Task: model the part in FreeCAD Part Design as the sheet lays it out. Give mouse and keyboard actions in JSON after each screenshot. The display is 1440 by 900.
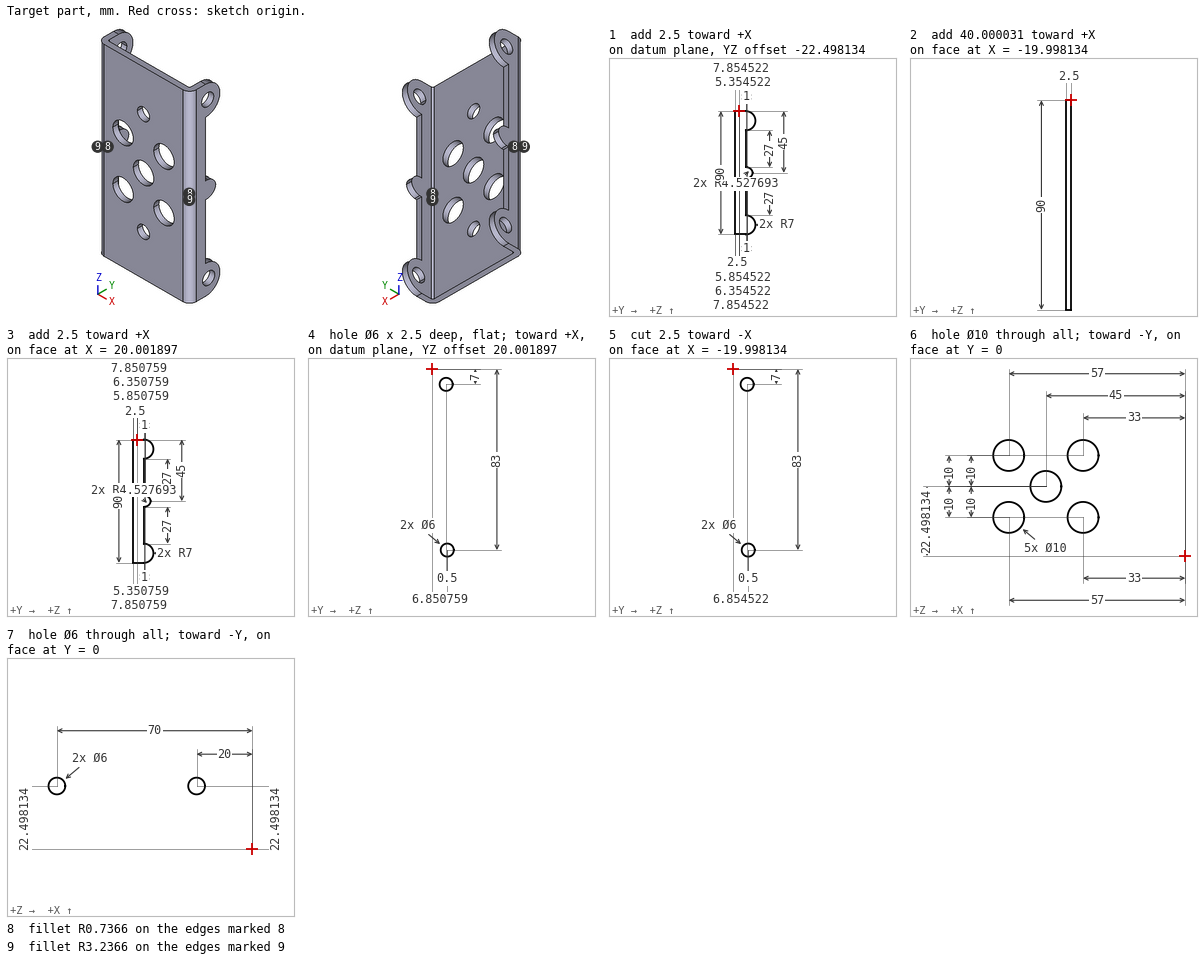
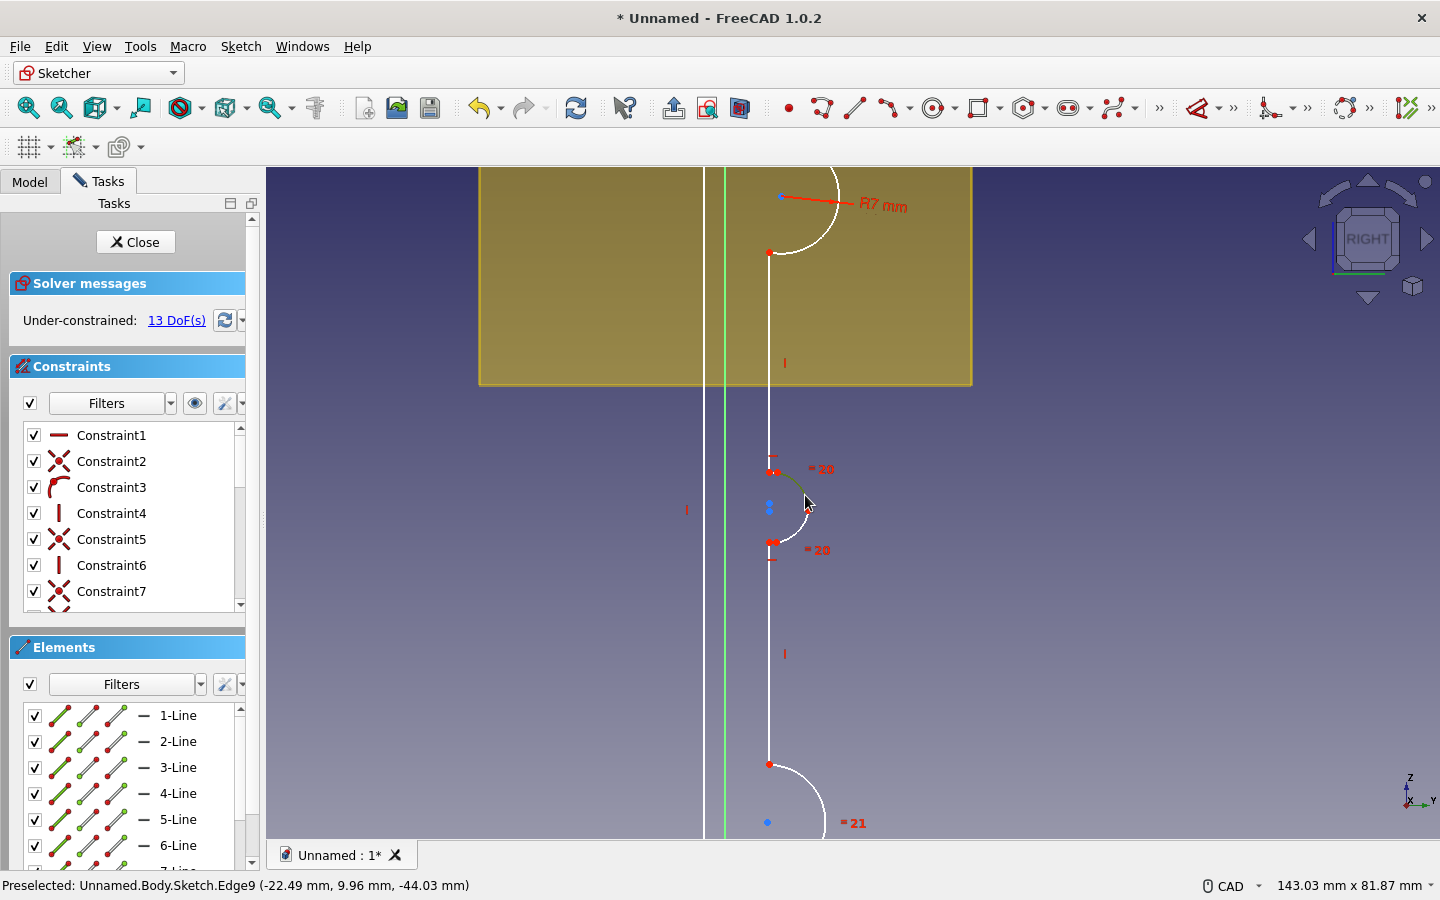
{"action": "left_click", "coordinate": [1218, 108]}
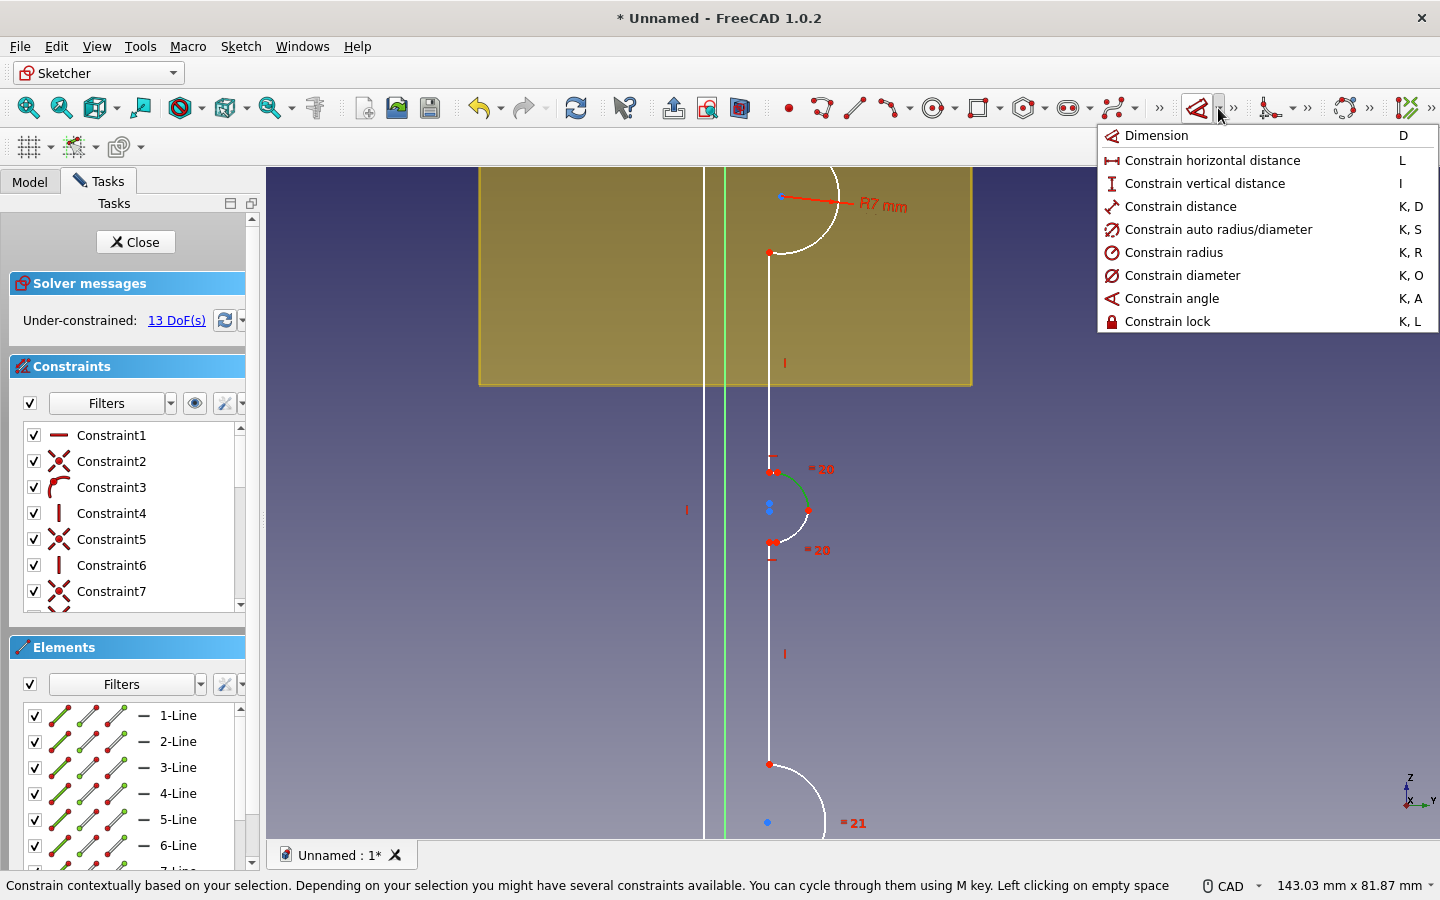
{"action": "left_click", "coordinate": [1268, 252]}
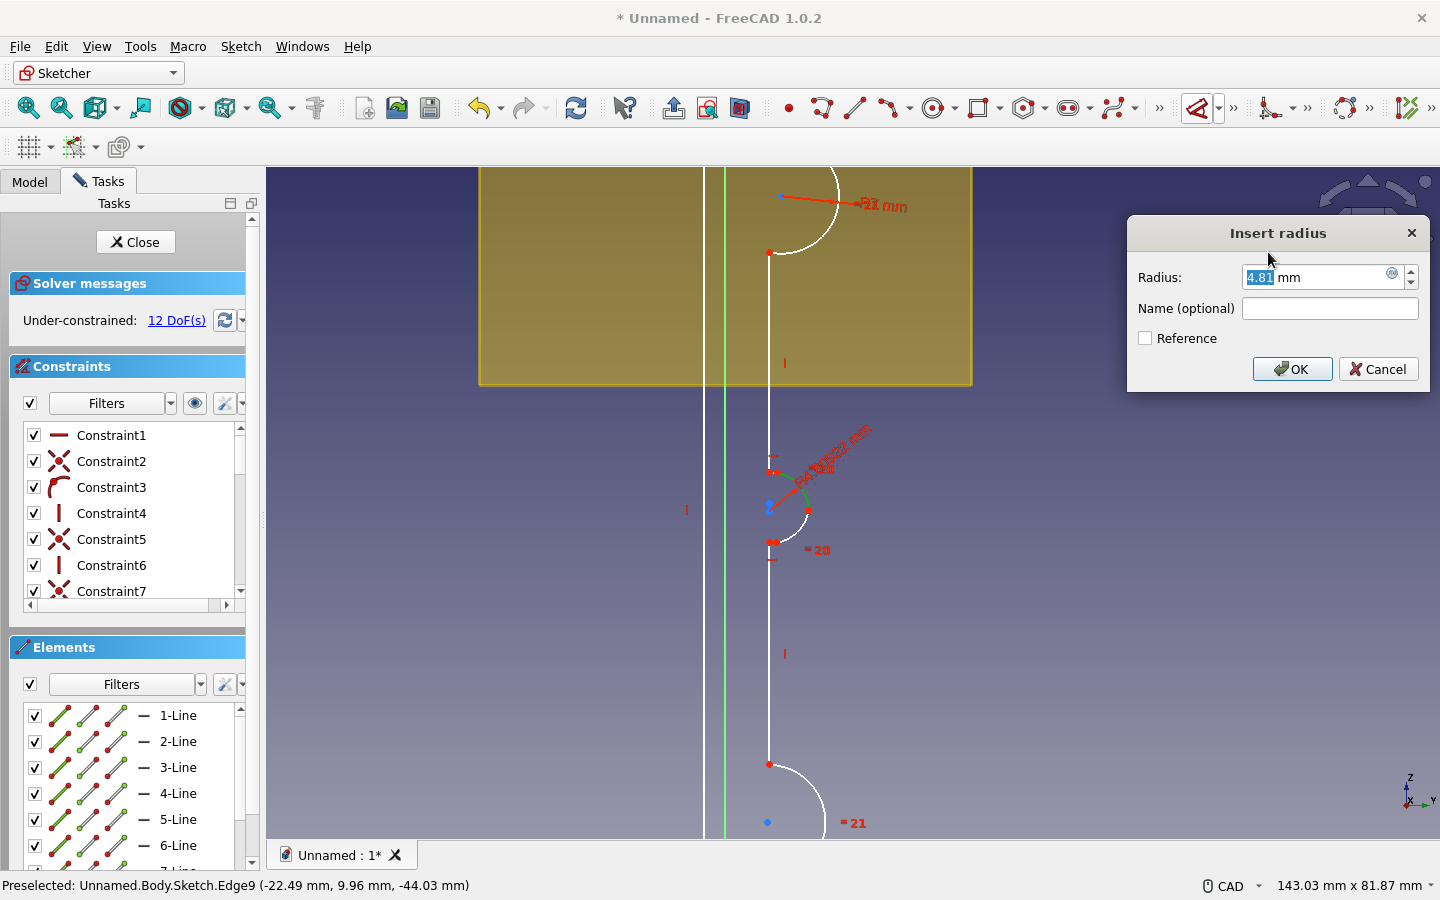
{"action": "type", "text": "4.527693"}
{"action": "key", "text": "Return"}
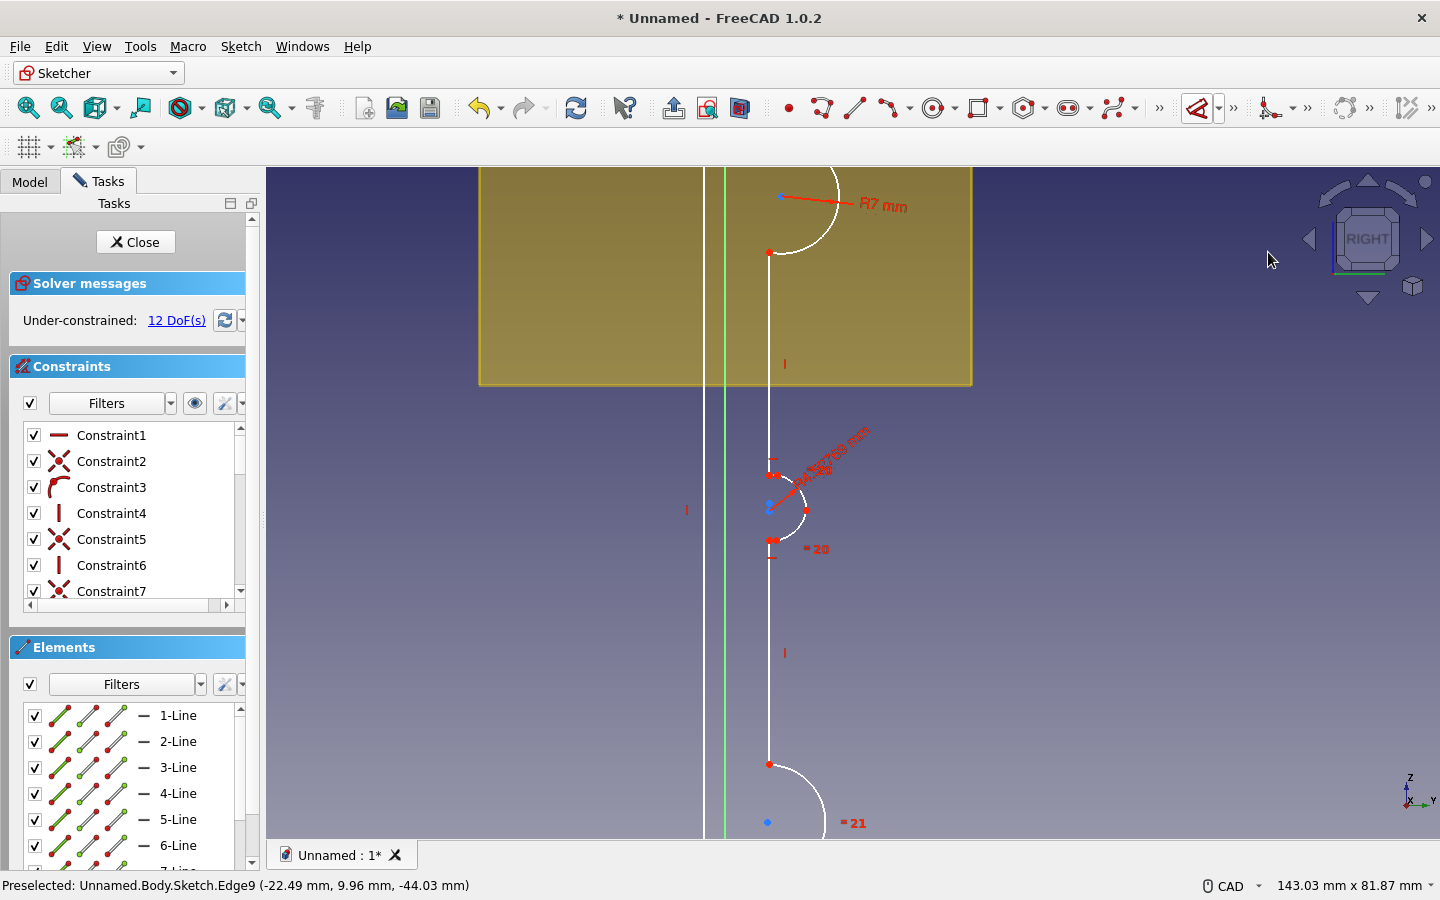
{"action": "scroll", "coordinate": [773, 475], "scroll_direction": "up", "scroll_amount": 8}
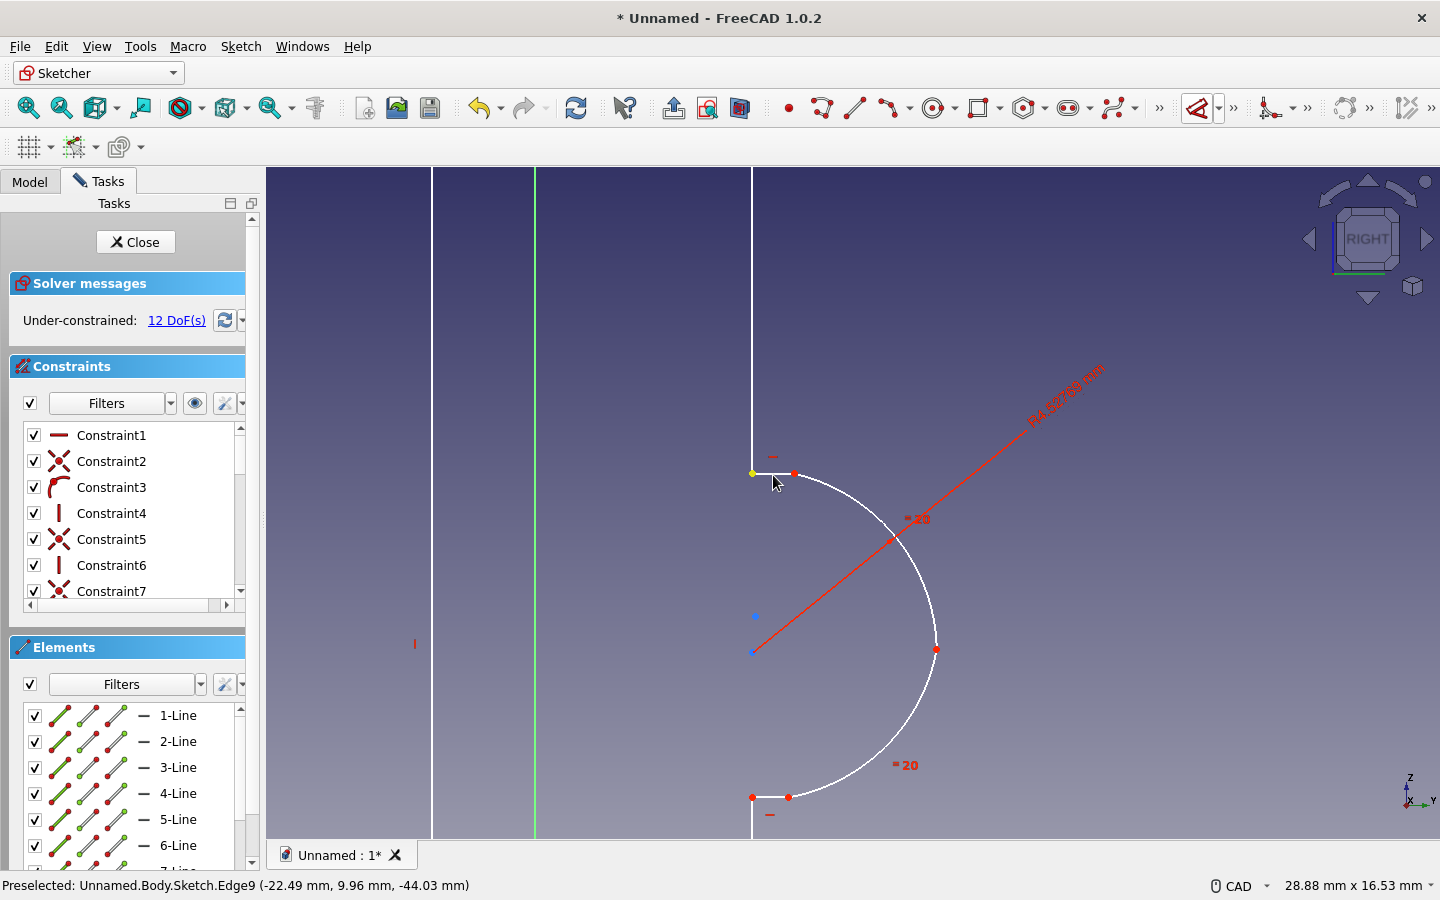
{"action": "left_click", "coordinate": [773, 474]}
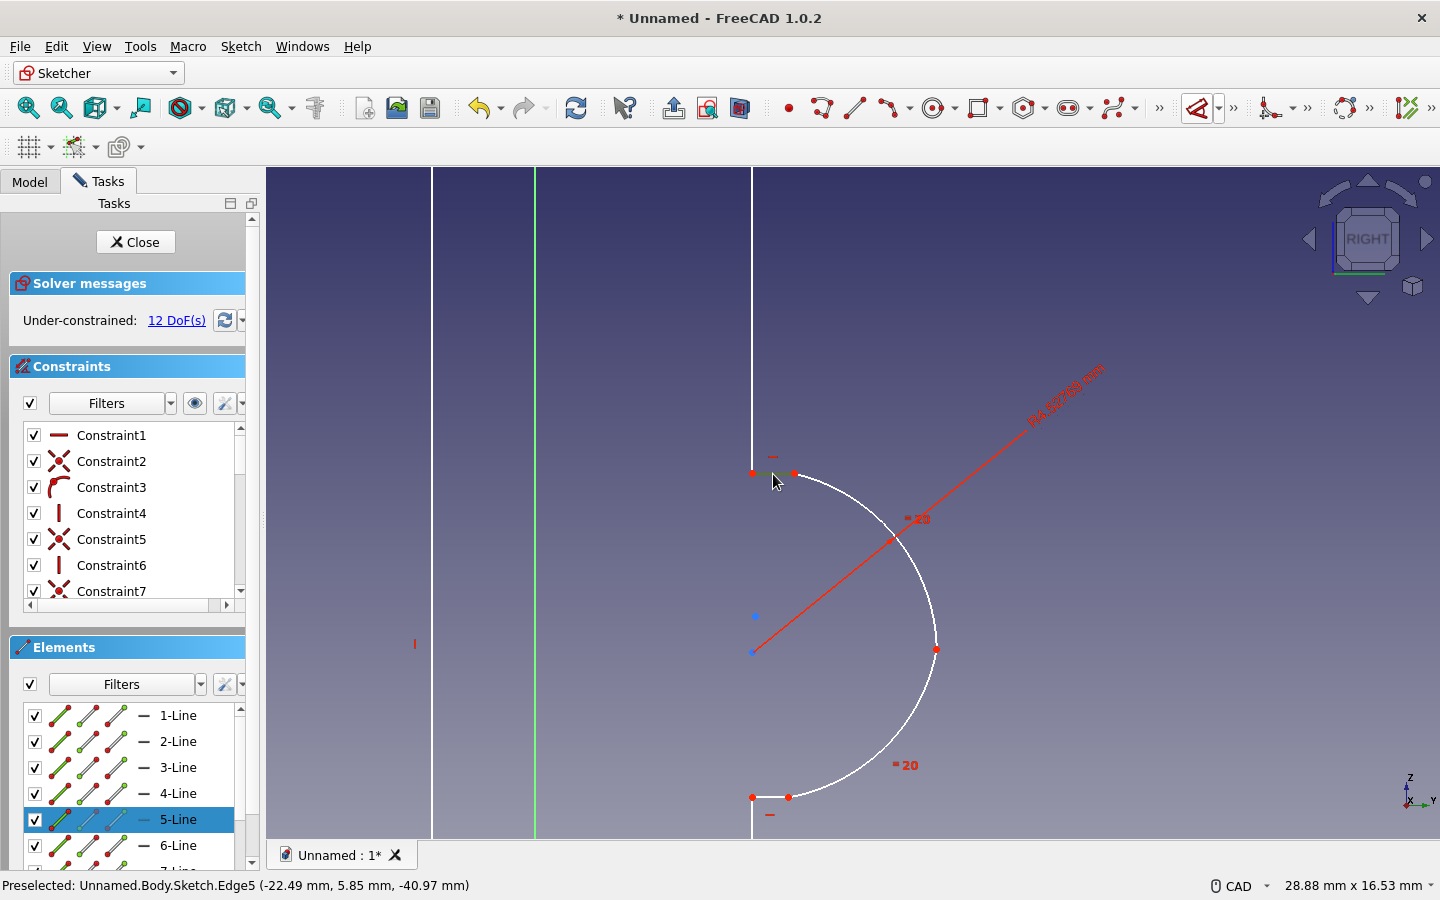
{"action": "left_click", "coordinate": [1218, 108]}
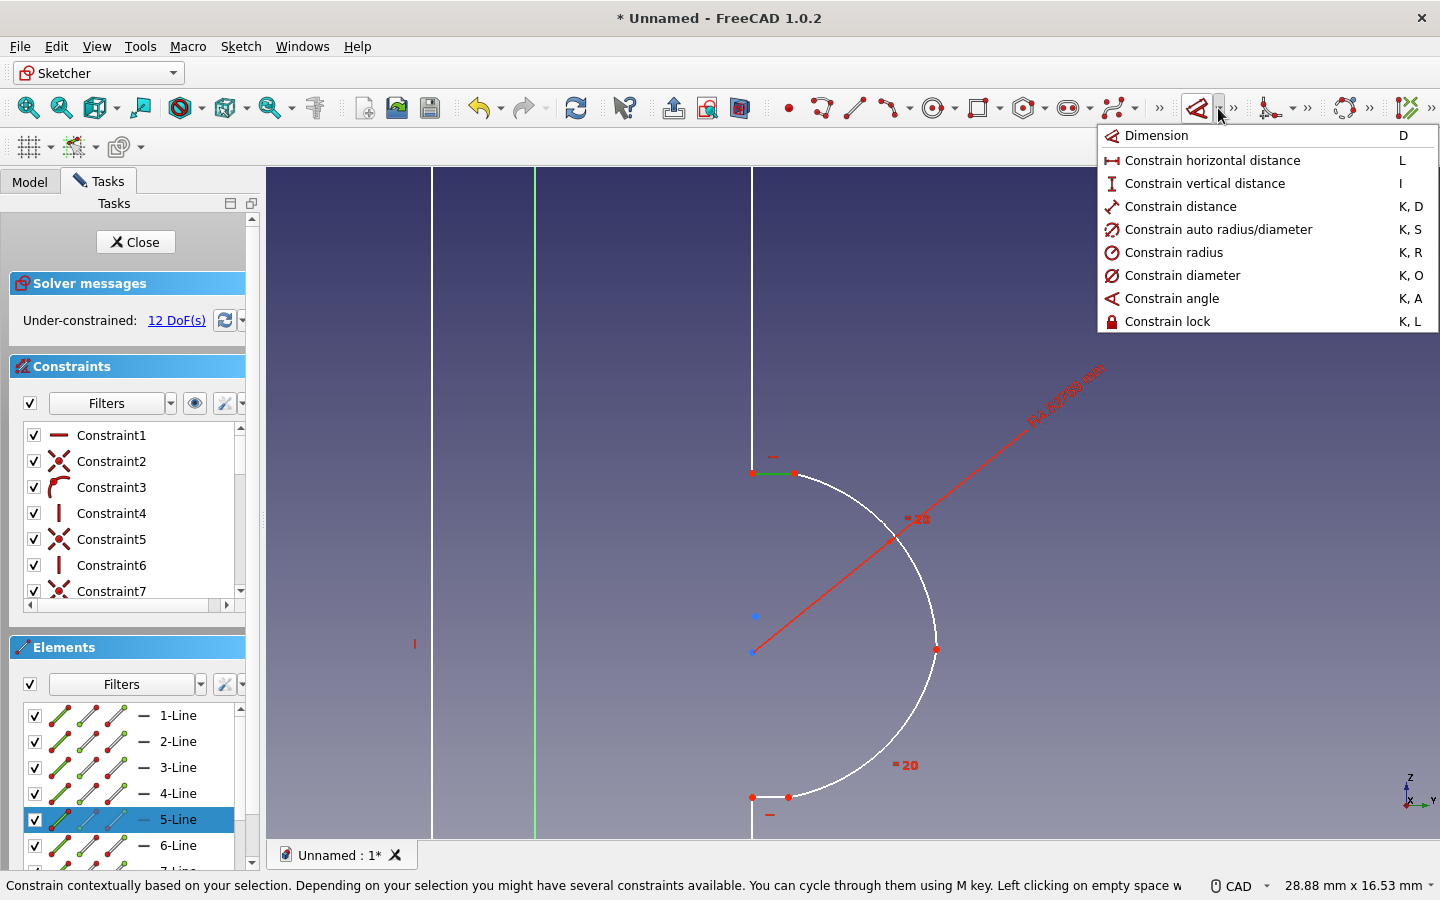
{"action": "left_click", "coordinate": [1268, 160]}